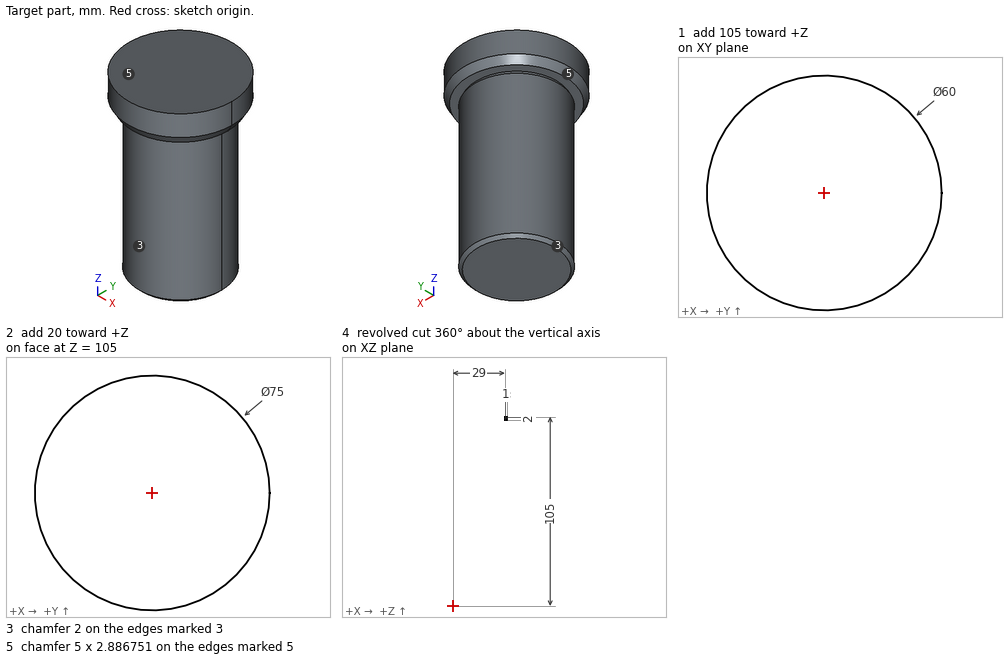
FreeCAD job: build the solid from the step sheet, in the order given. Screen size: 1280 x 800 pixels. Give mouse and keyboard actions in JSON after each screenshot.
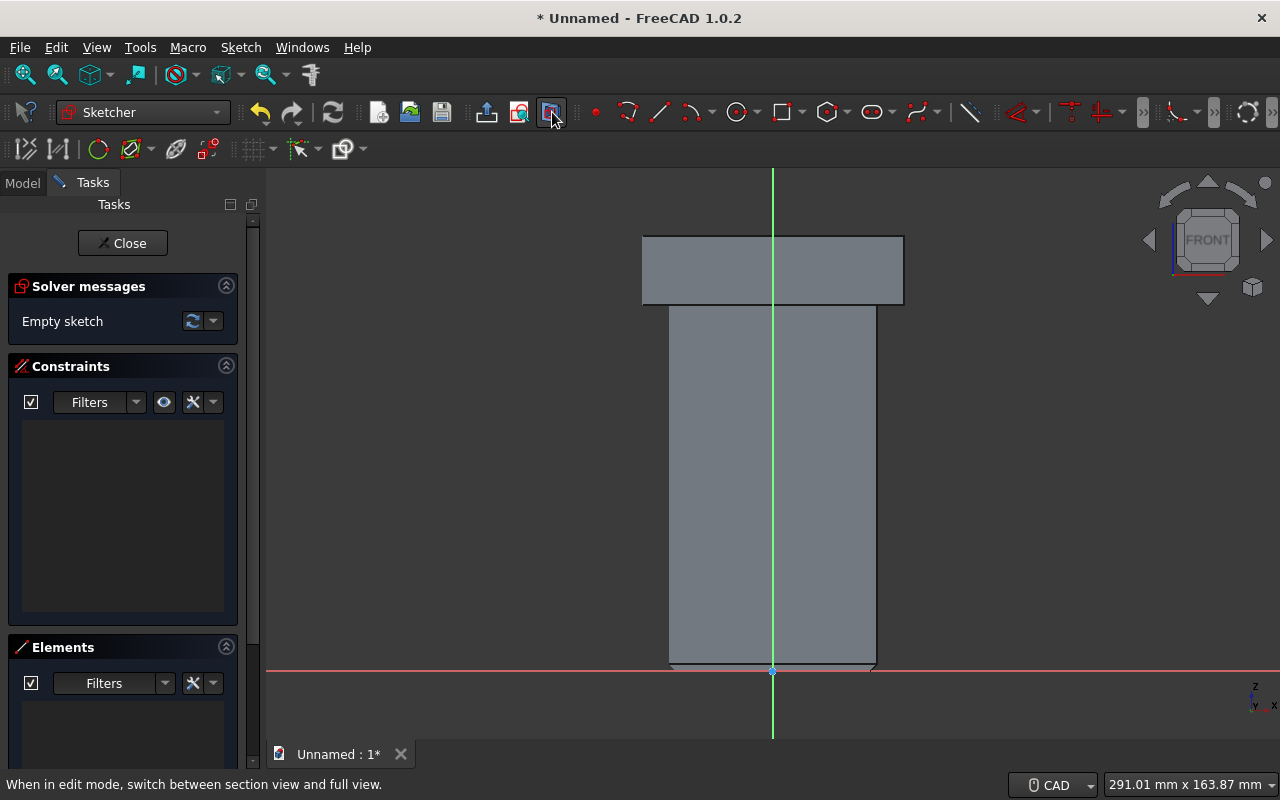
{"action": "scroll", "coordinate": [885, 301], "scroll_direction": "up", "scroll_amount": 15}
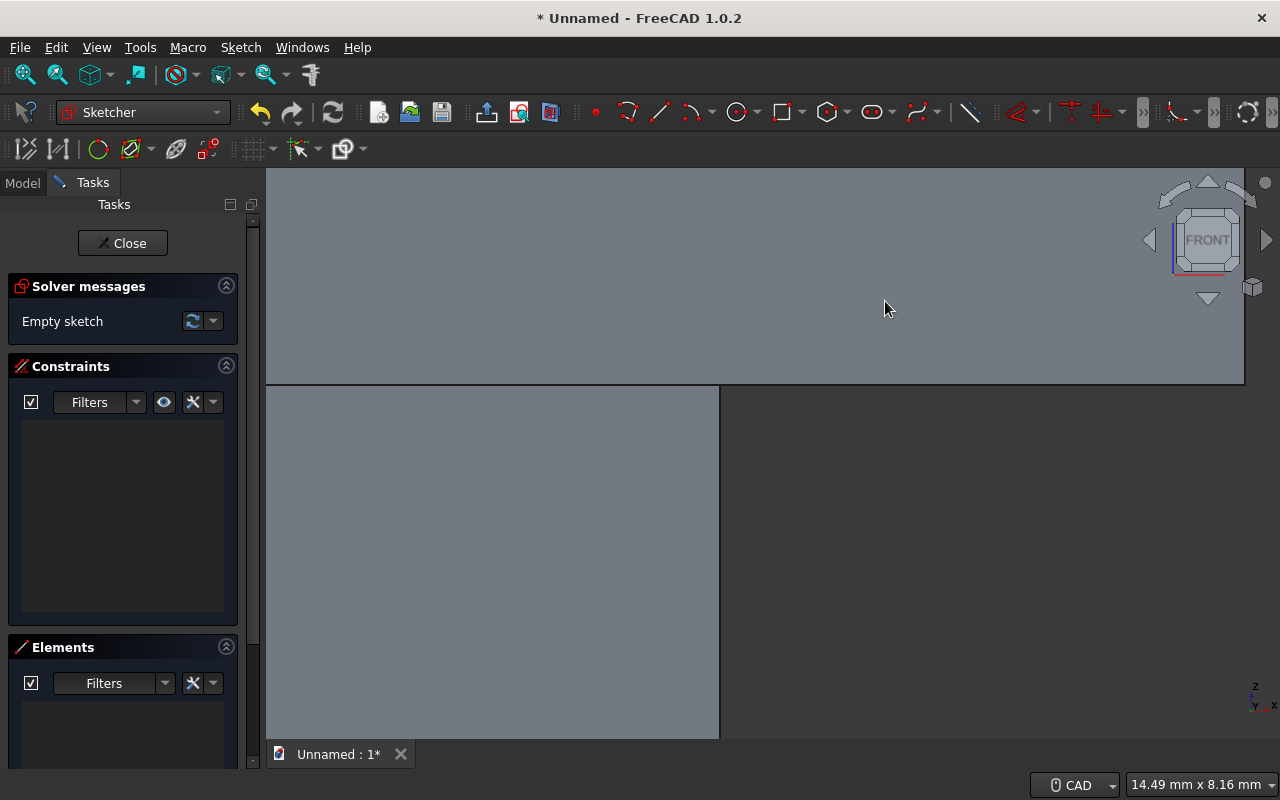
{"action": "scroll", "coordinate": [674, 456], "scroll_direction": "up", "scroll_amount": 5}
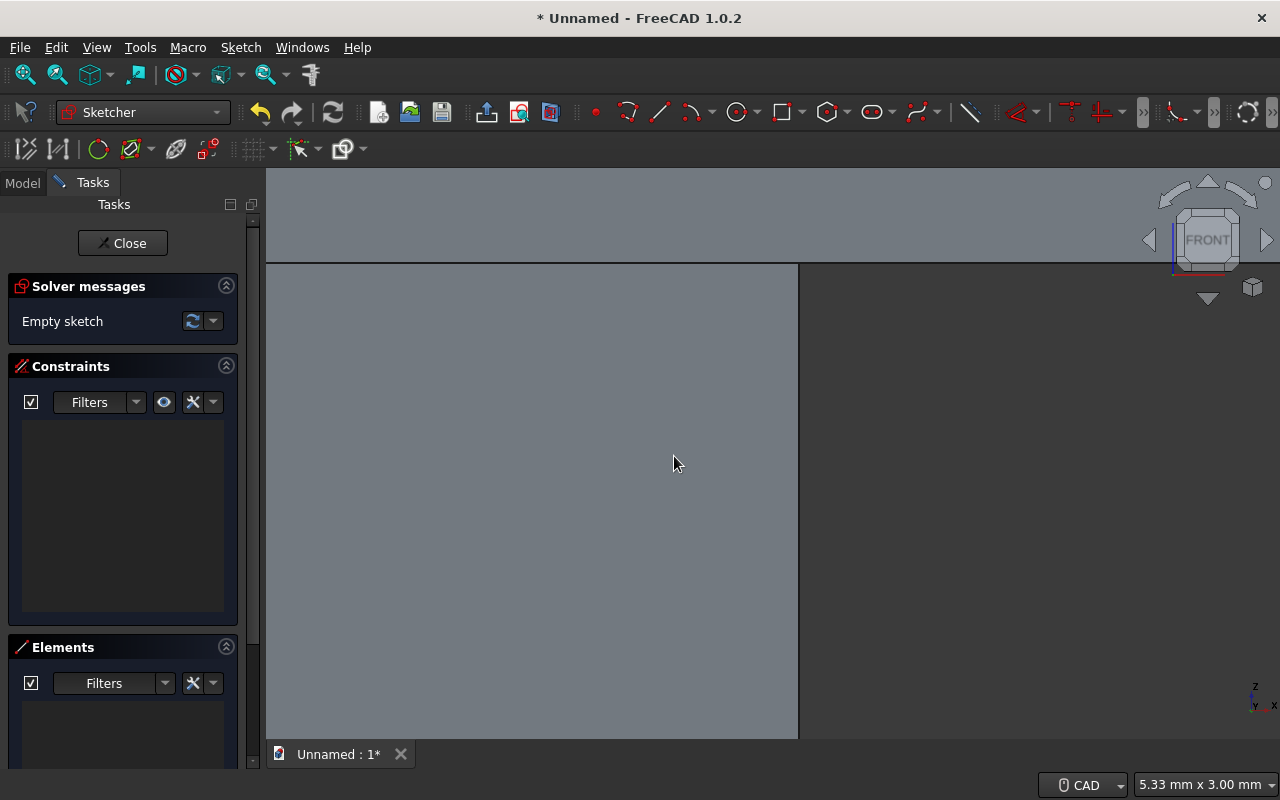
{"action": "left_click", "coordinate": [782, 112]}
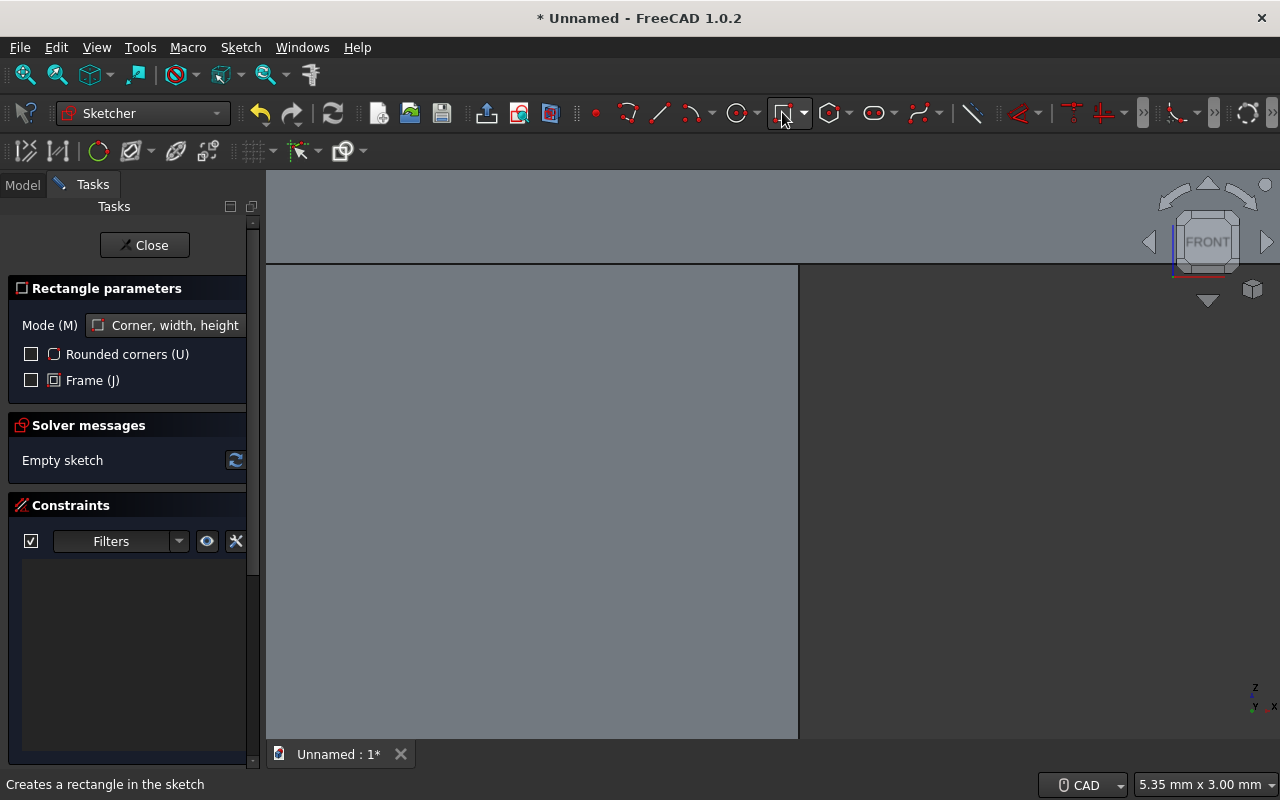
{"action": "left_click", "coordinate": [609, 264]}
{"action": "mouse_move", "coordinate": [799, 643]}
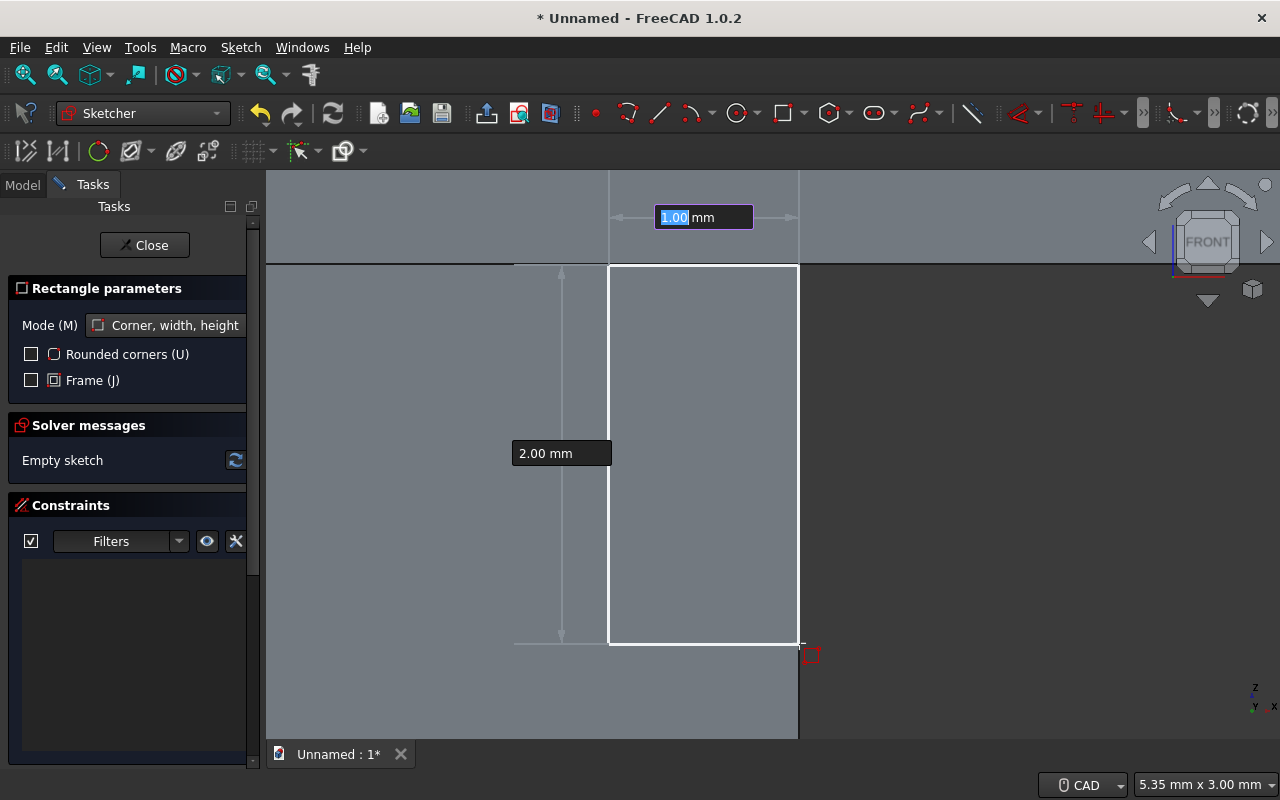
{"action": "type", "text": "1"}
{"action": "key", "text": "Tab"}
{"action": "type", "text": "2"}
{"action": "key", "text": "Return"}
{"action": "key", "text": "Escape"}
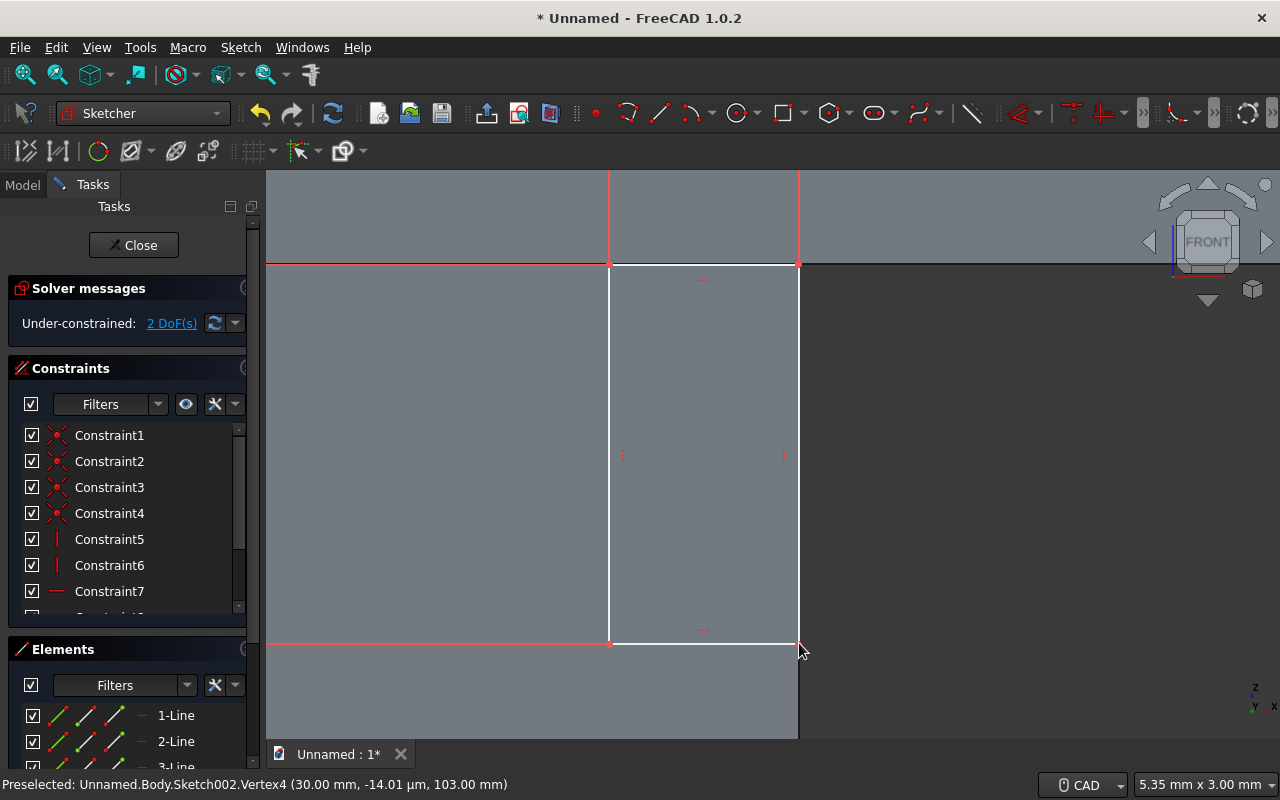
{"action": "left_click", "coordinate": [1018, 114]}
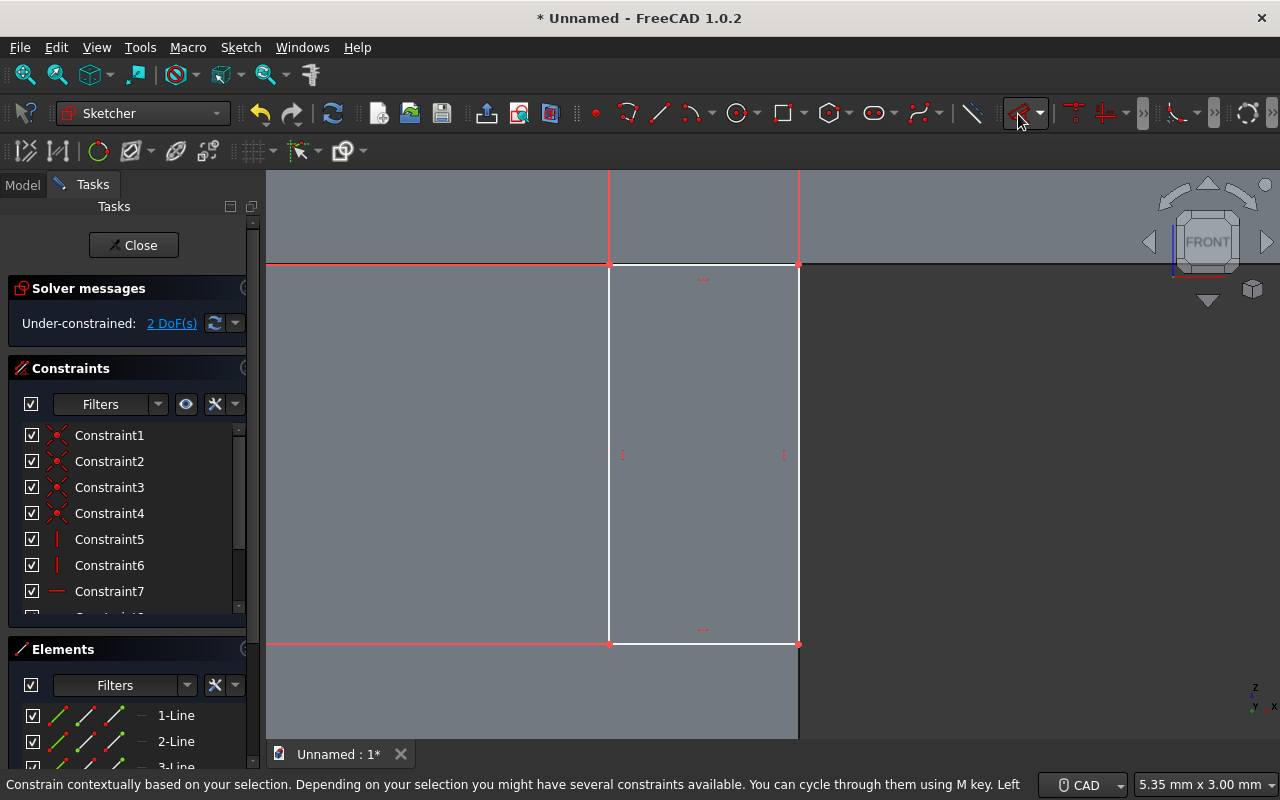
{"action": "left_click", "coordinate": [609, 265]}
{"action": "left_click", "coordinate": [452, 231]}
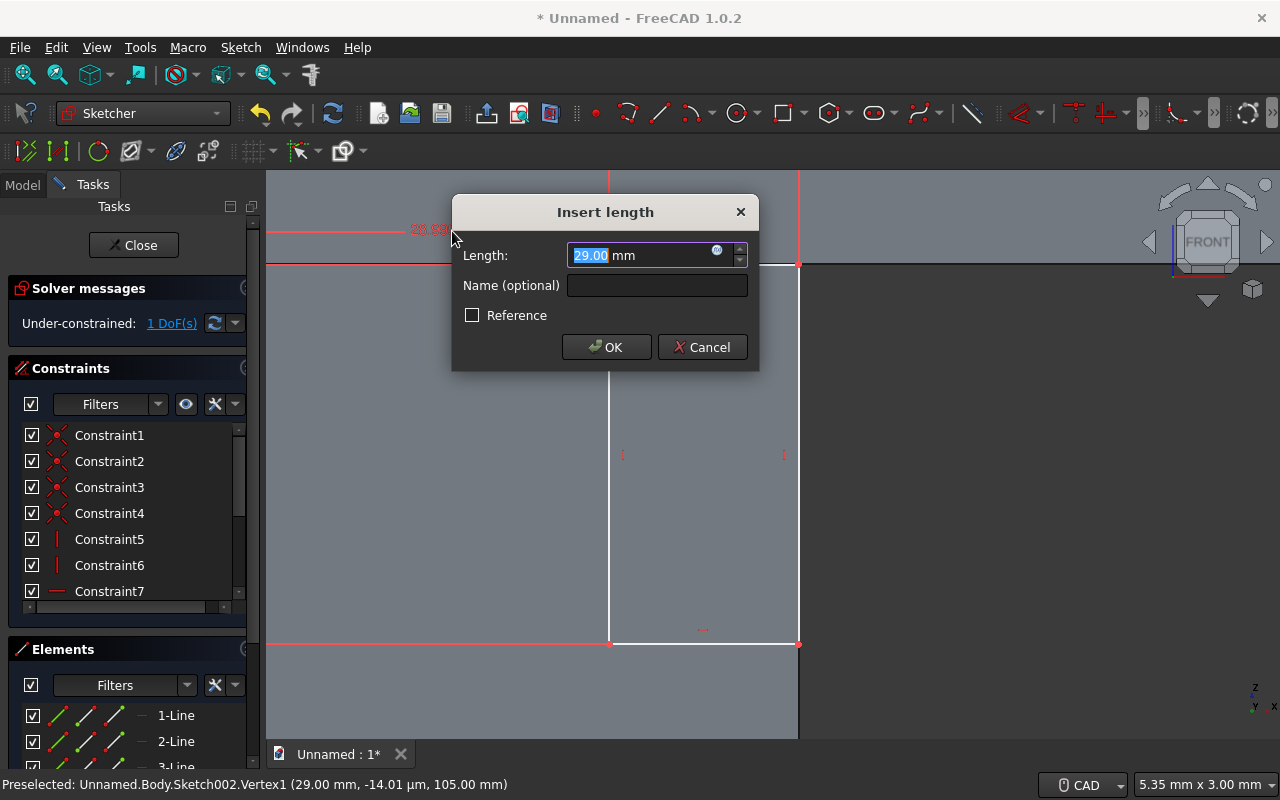
{"action": "type", "text": "29"}
{"action": "key", "text": "Return"}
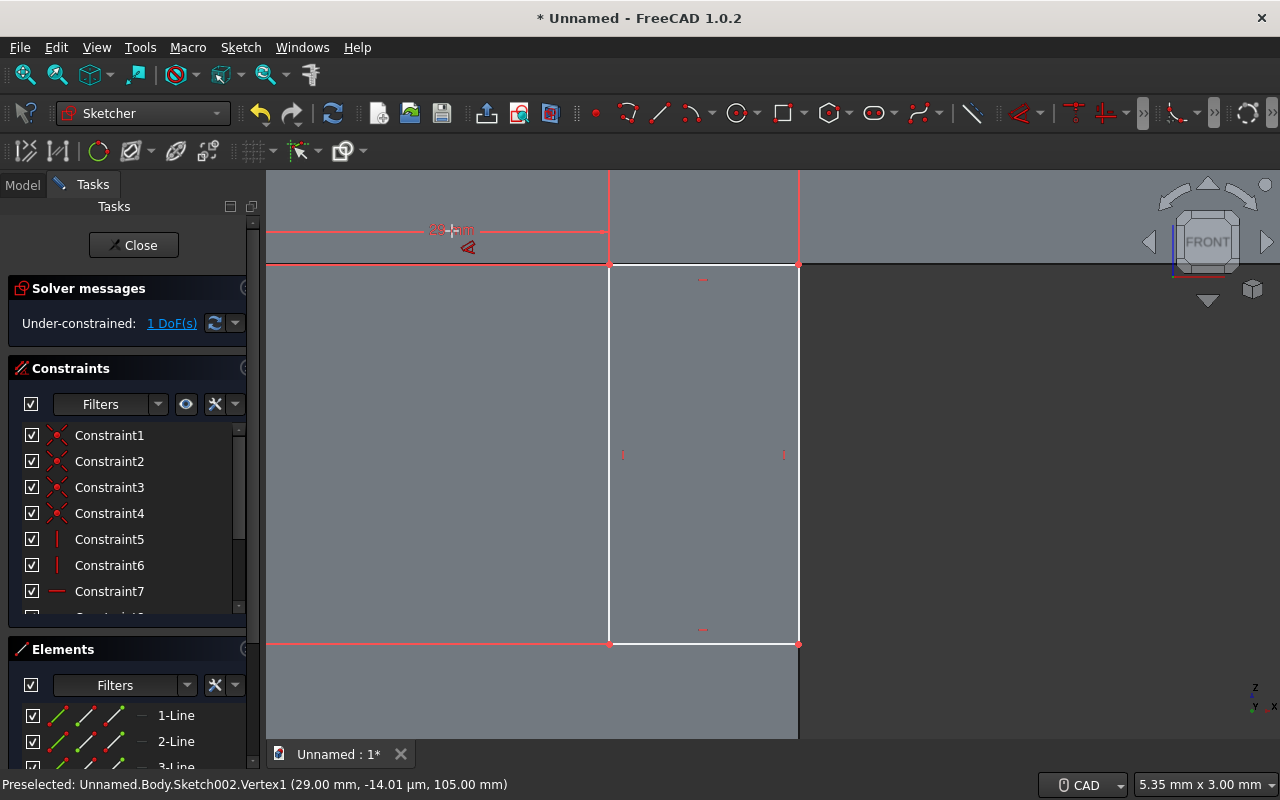
{"action": "left_click", "coordinate": [609, 265]}
{"action": "left_click", "coordinate": [643, 488]}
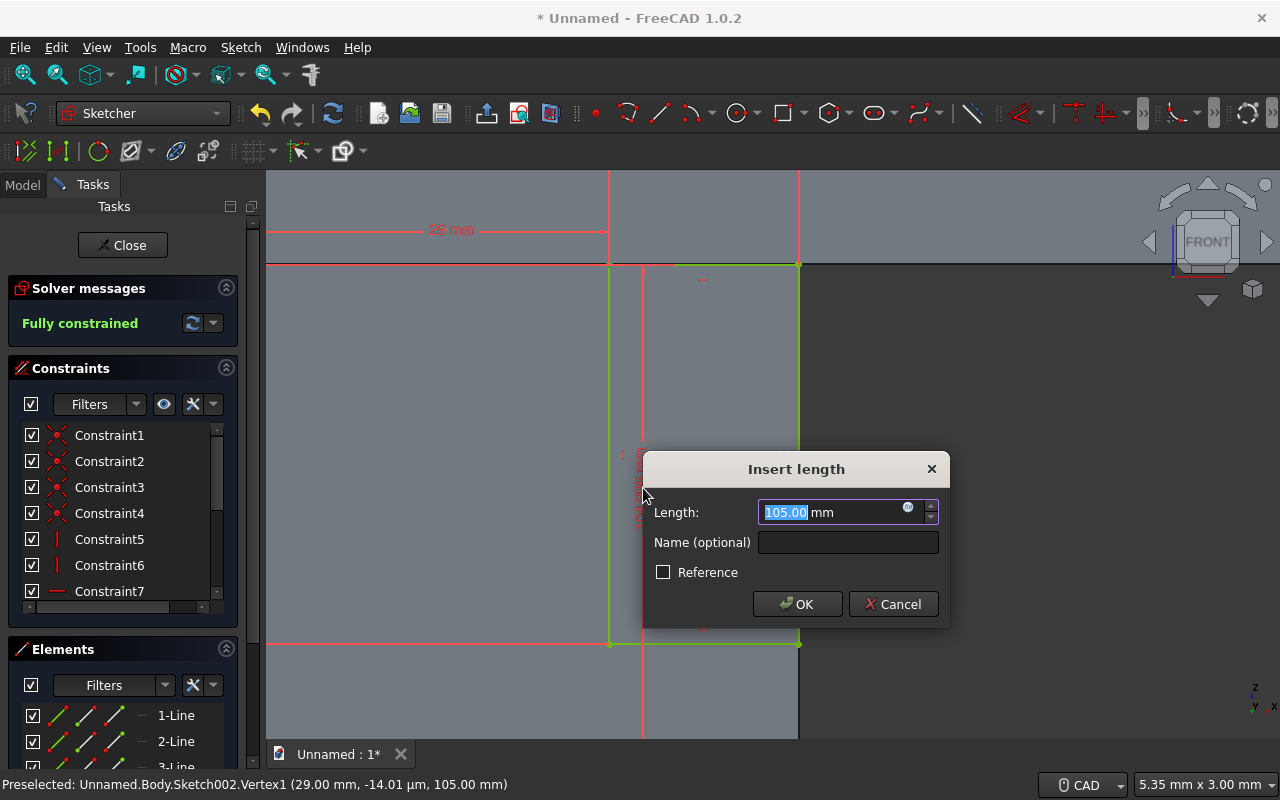
{"action": "type", "text": "105"}
{"action": "key", "text": "Return"}
{"action": "key", "text": "Escape"}